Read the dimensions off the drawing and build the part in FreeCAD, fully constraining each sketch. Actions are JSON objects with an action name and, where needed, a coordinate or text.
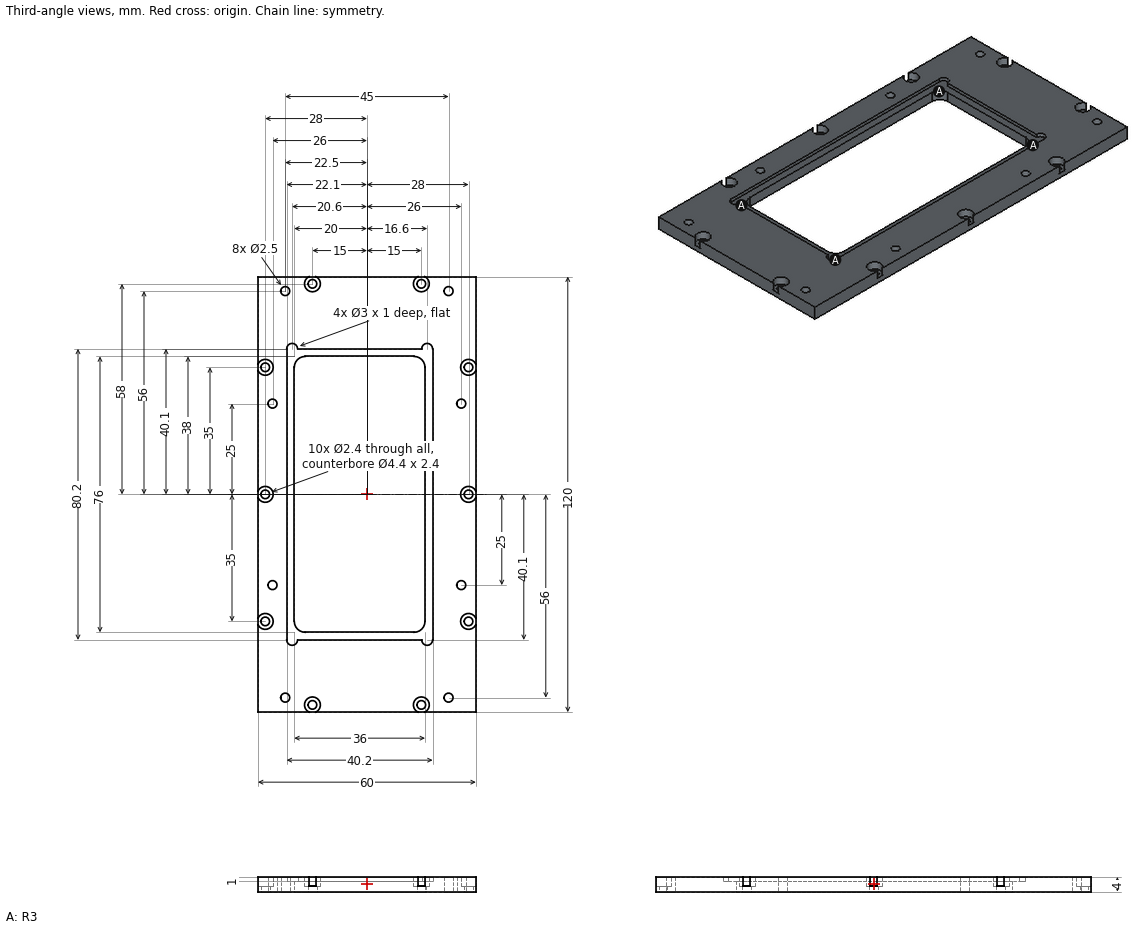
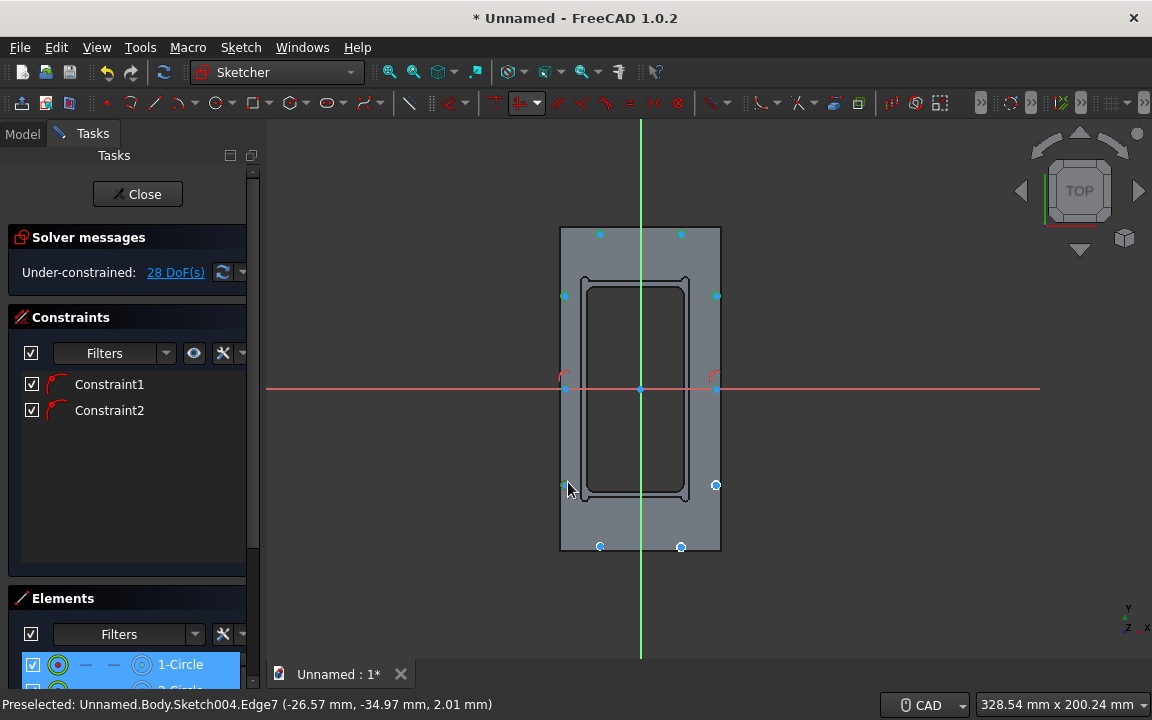
{"action": "scroll", "coordinate": [719, 482], "scroll_direction": "up", "scroll_amount": 6}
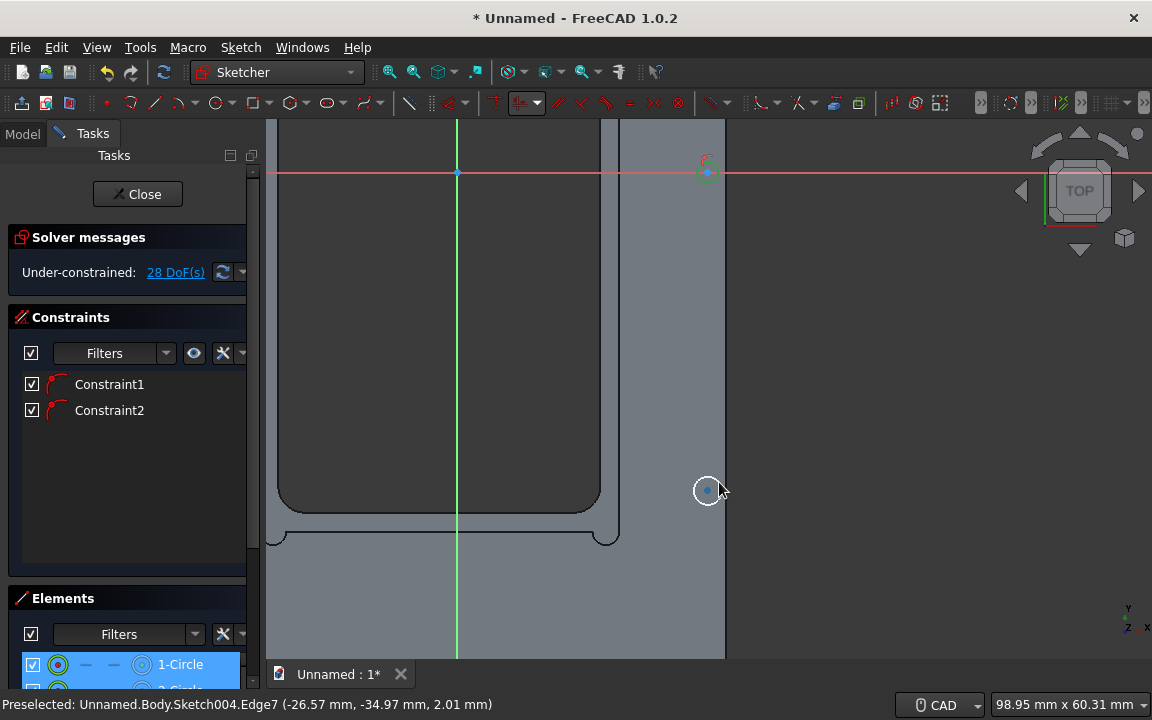
{"action": "left_click", "coordinate": [718, 481]}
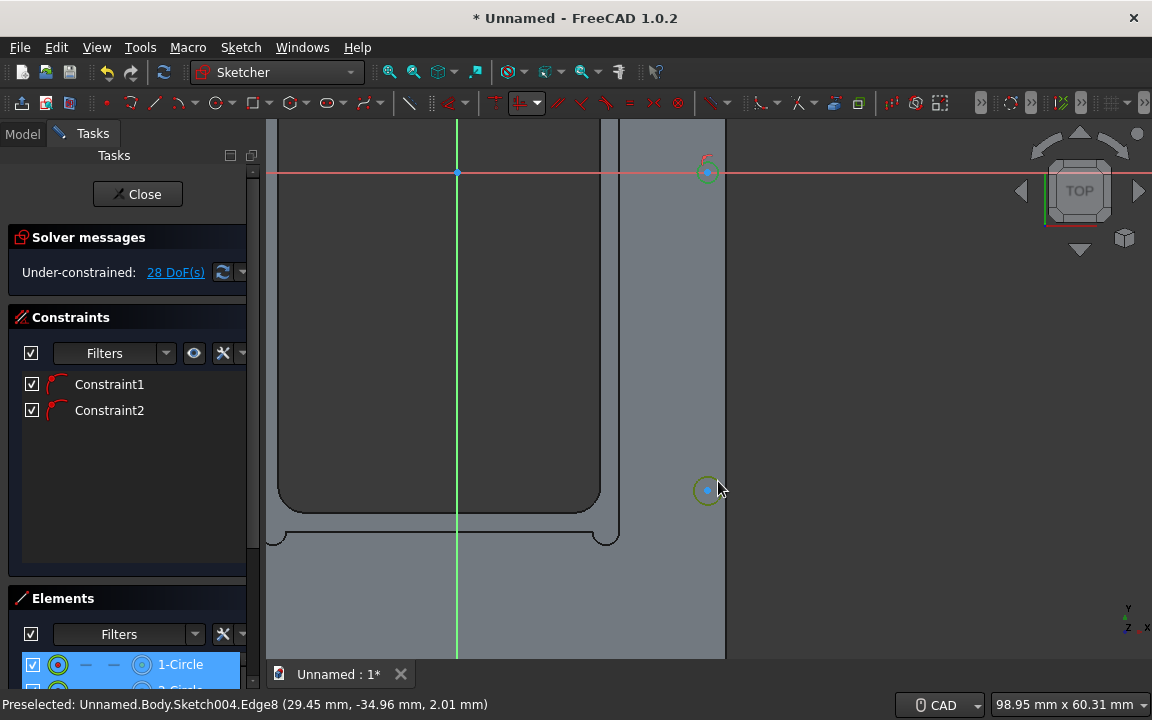
{"action": "scroll", "coordinate": [719, 482], "scroll_direction": "down", "scroll_amount": 6}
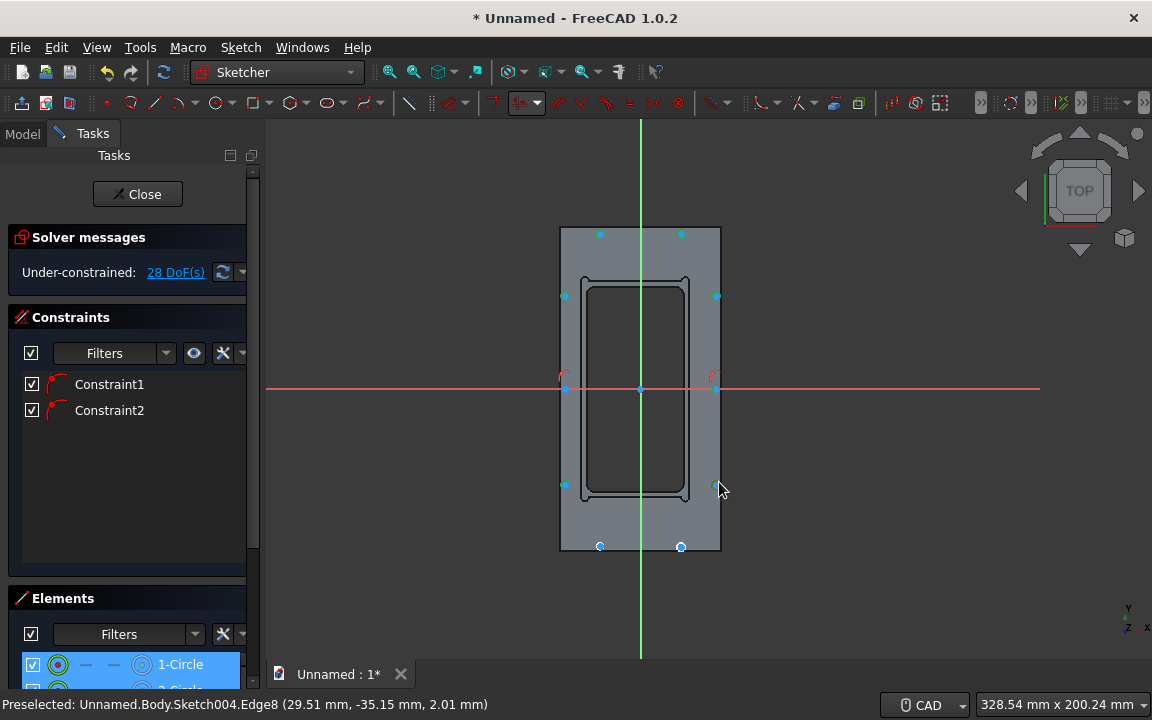
{"action": "scroll", "coordinate": [602, 544], "scroll_direction": "up", "scroll_amount": 7}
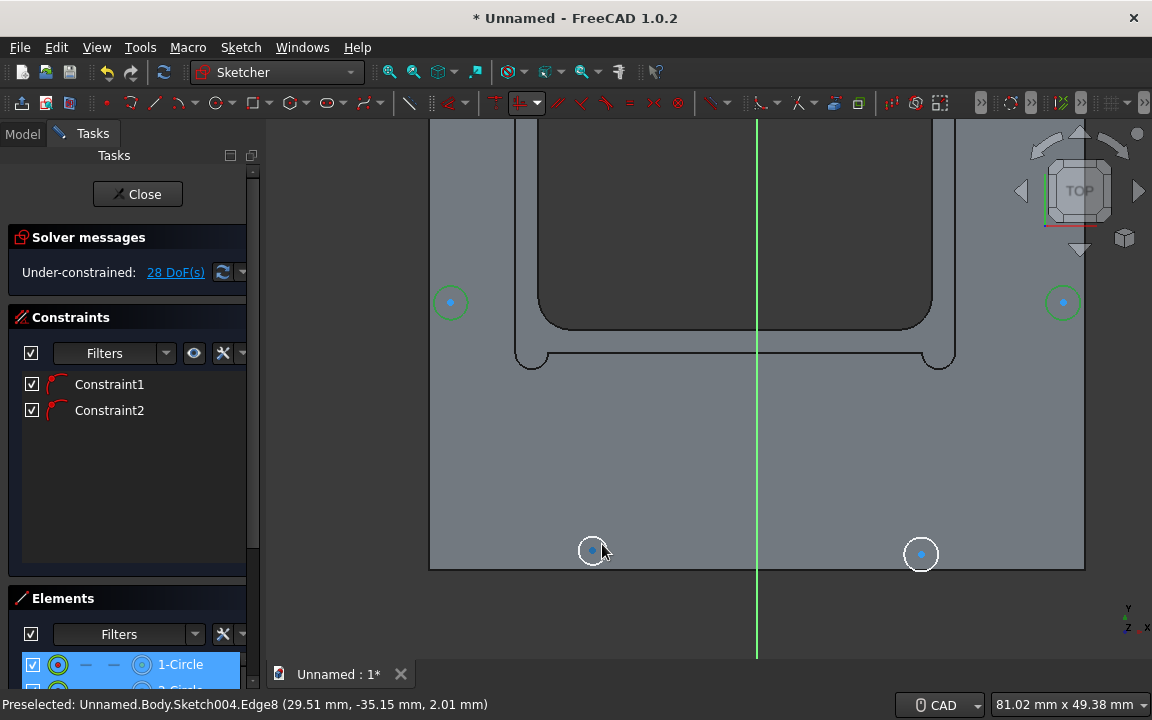
{"action": "left_click", "coordinate": [603, 541]}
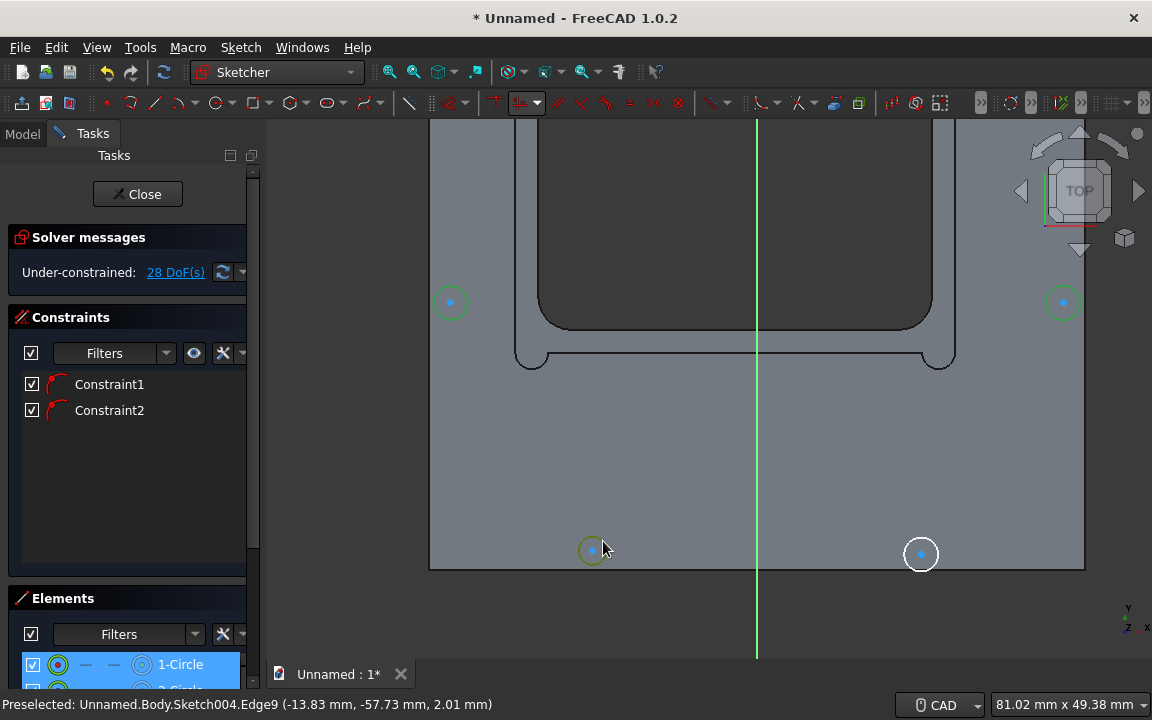
{"action": "left_click", "coordinate": [933, 543]}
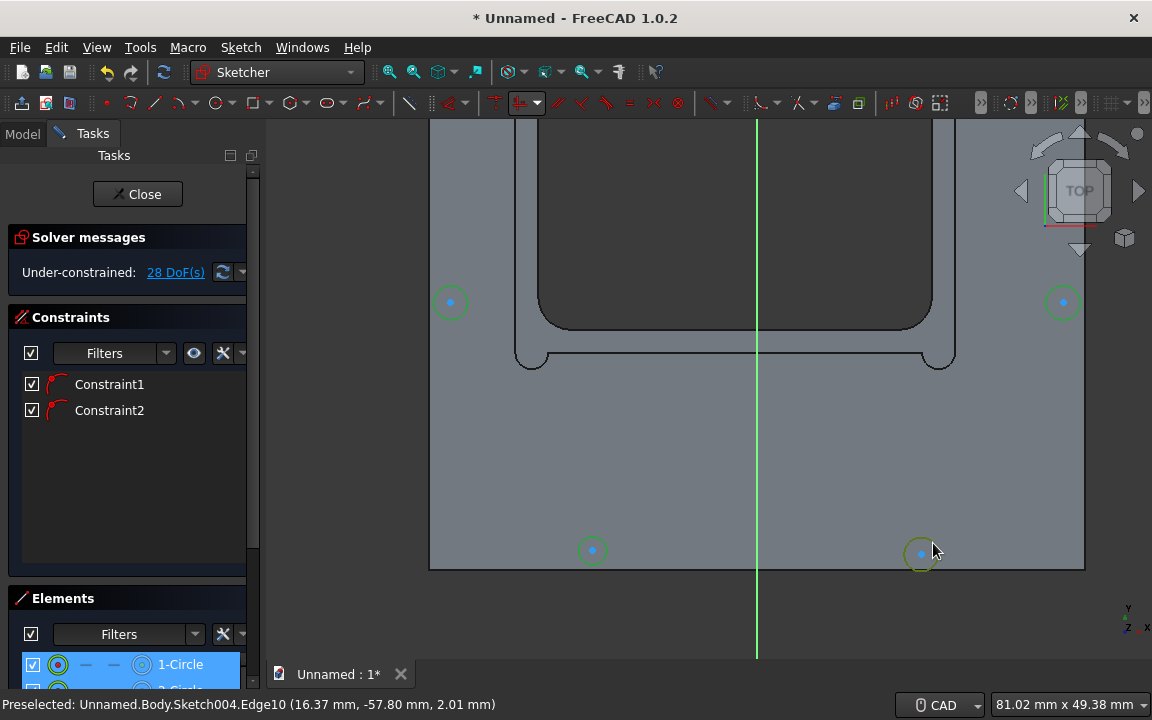
{"action": "left_click", "coordinate": [630, 104]}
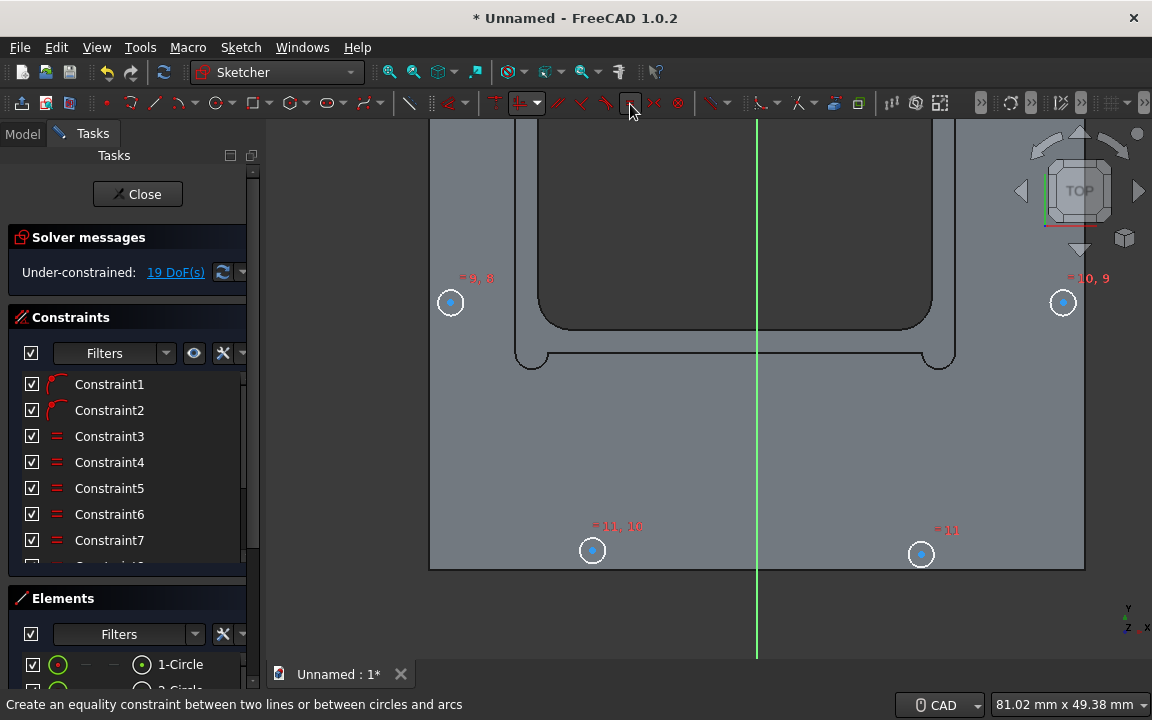
{"action": "scroll", "coordinate": [602, 544], "scroll_direction": "down", "scroll_amount": 7}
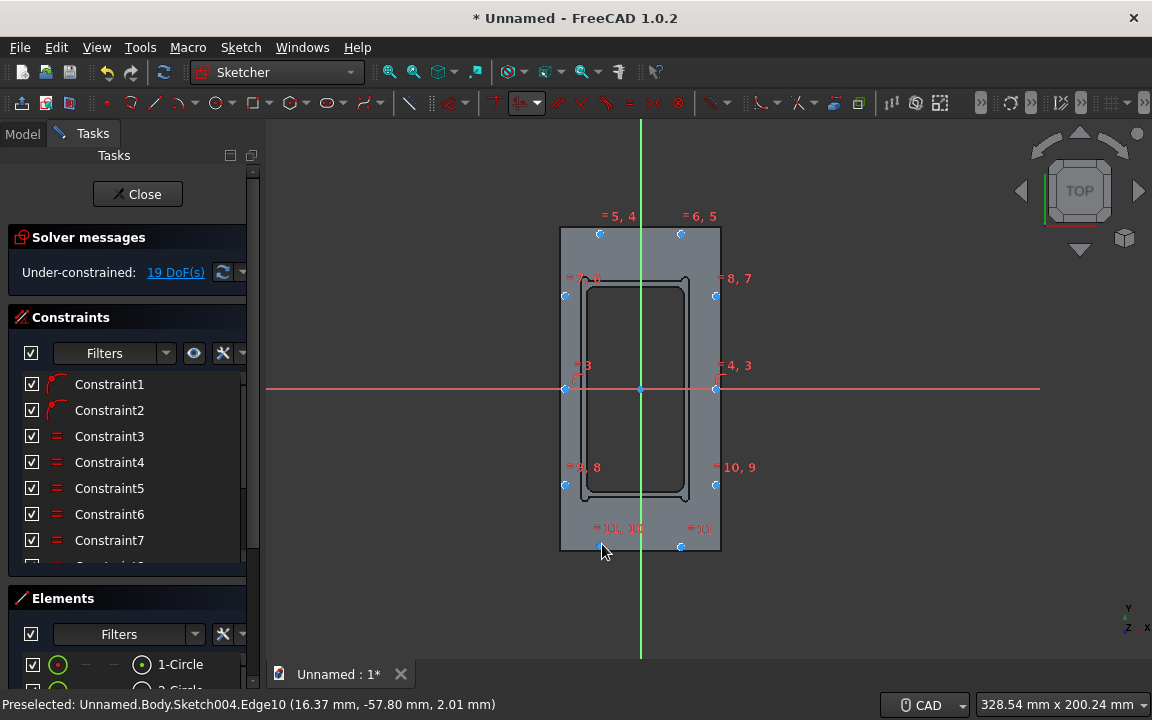
{"action": "left_click", "coordinate": [600, 234]}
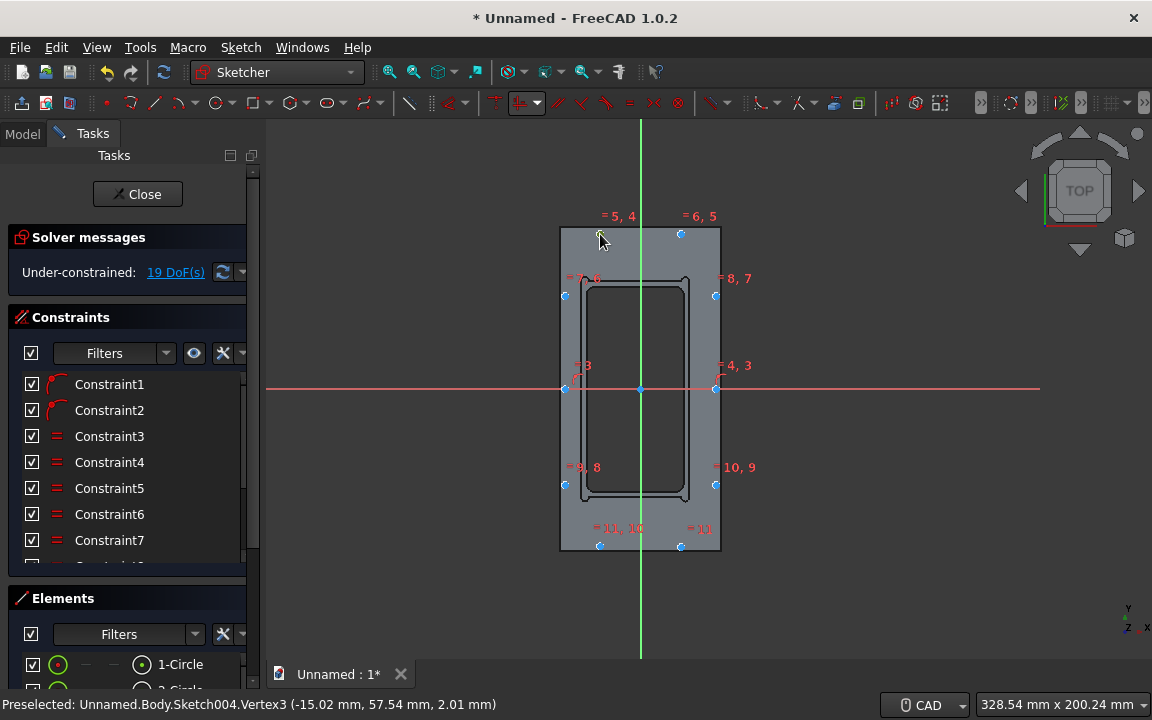
{"action": "left_click", "coordinate": [681, 234]}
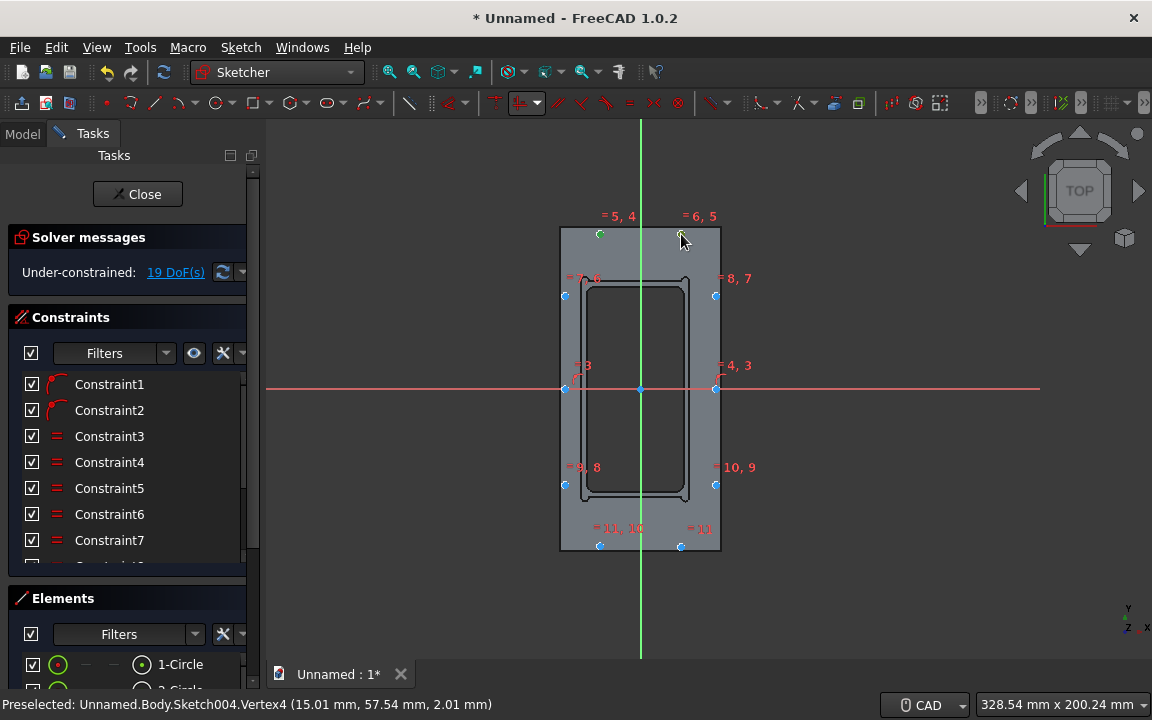
{"action": "key", "text": "h"}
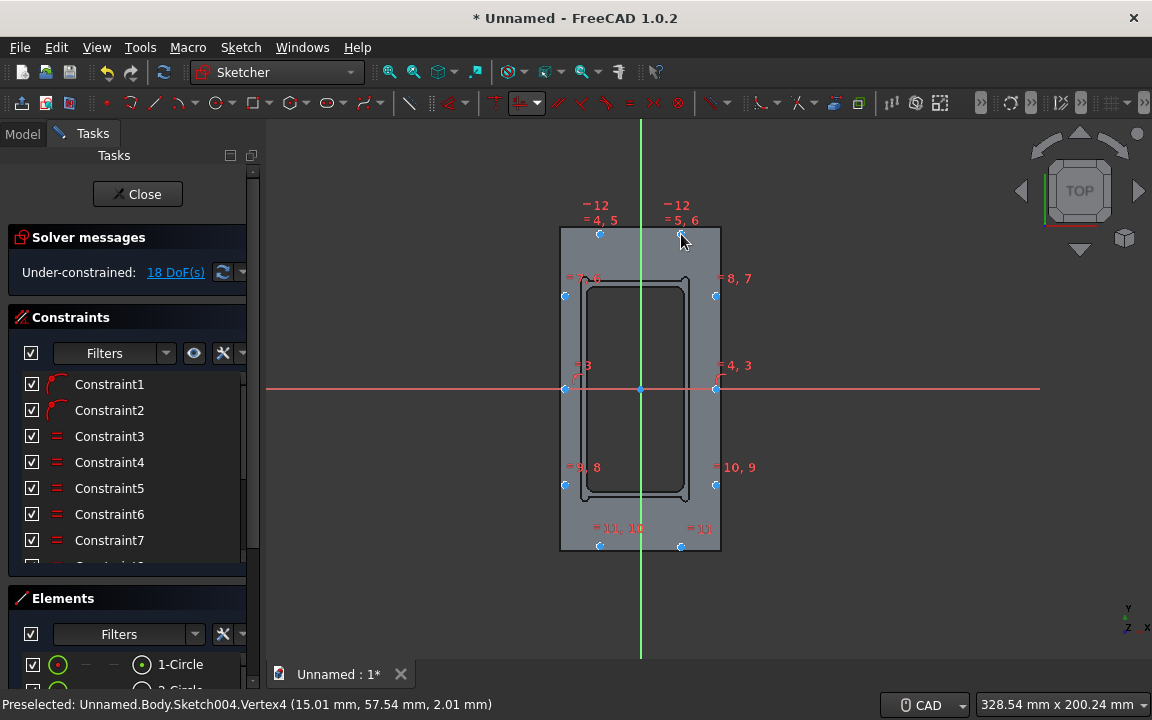
{"action": "left_click", "coordinate": [565, 389]}